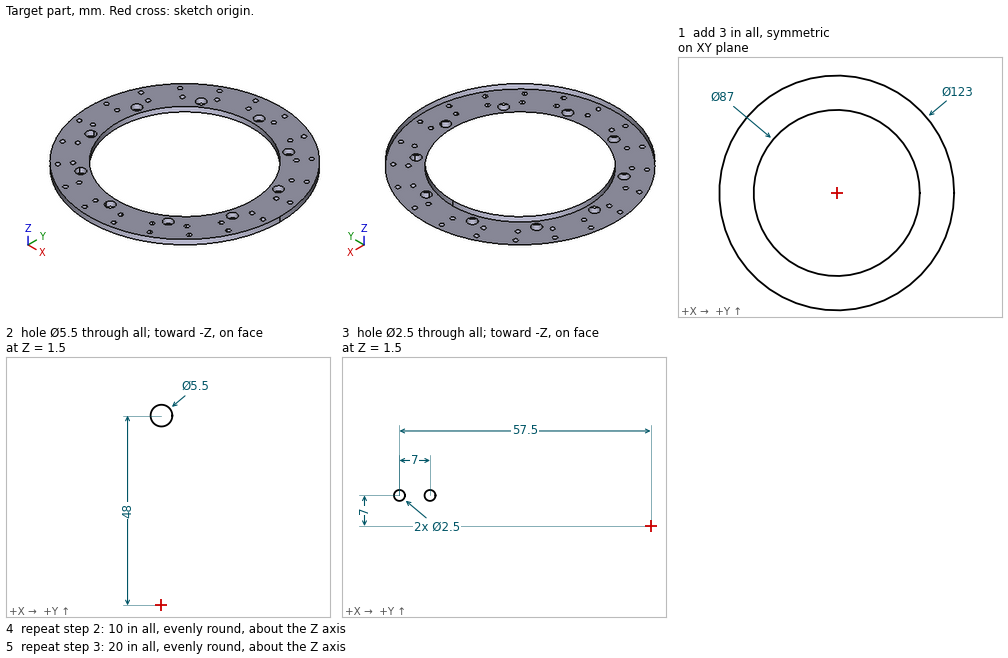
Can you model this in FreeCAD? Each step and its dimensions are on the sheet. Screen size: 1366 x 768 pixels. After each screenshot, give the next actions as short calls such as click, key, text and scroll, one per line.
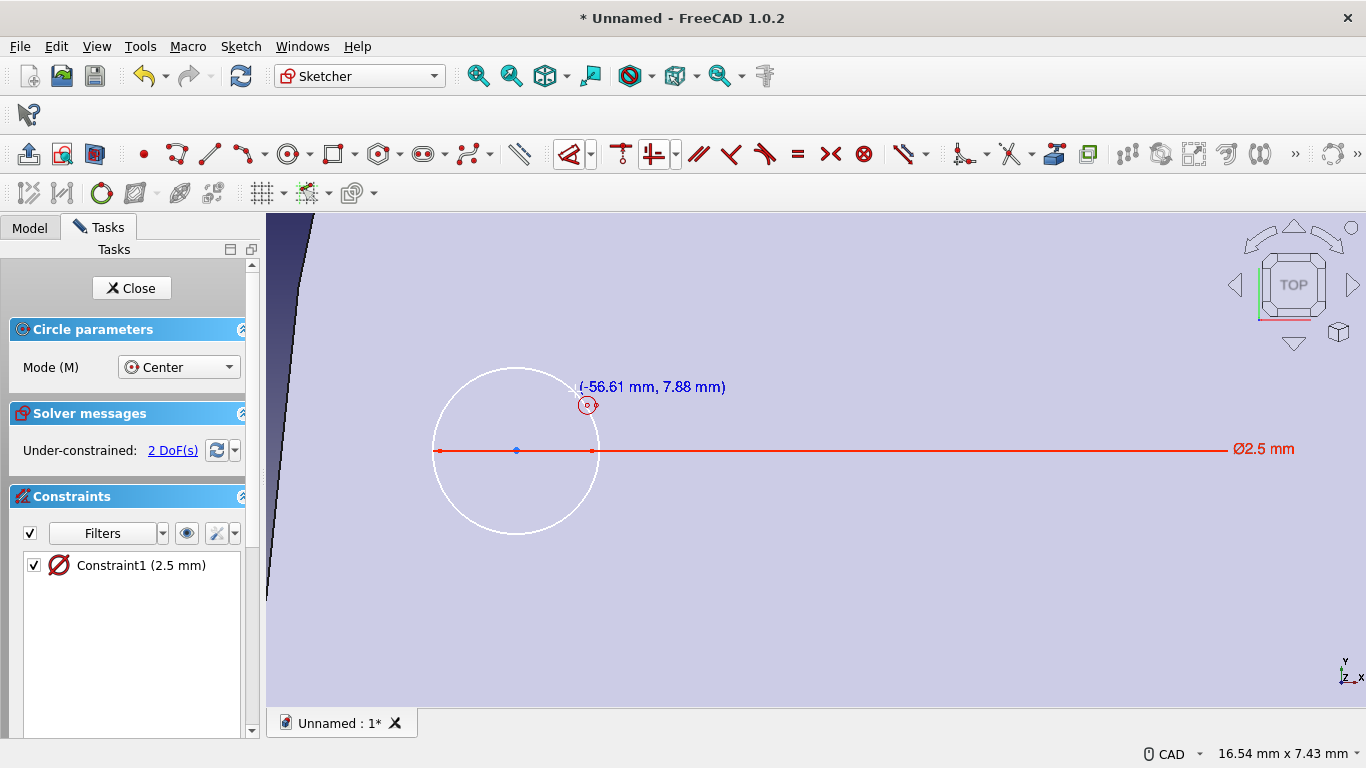
click(981, 450)
move(1040, 391)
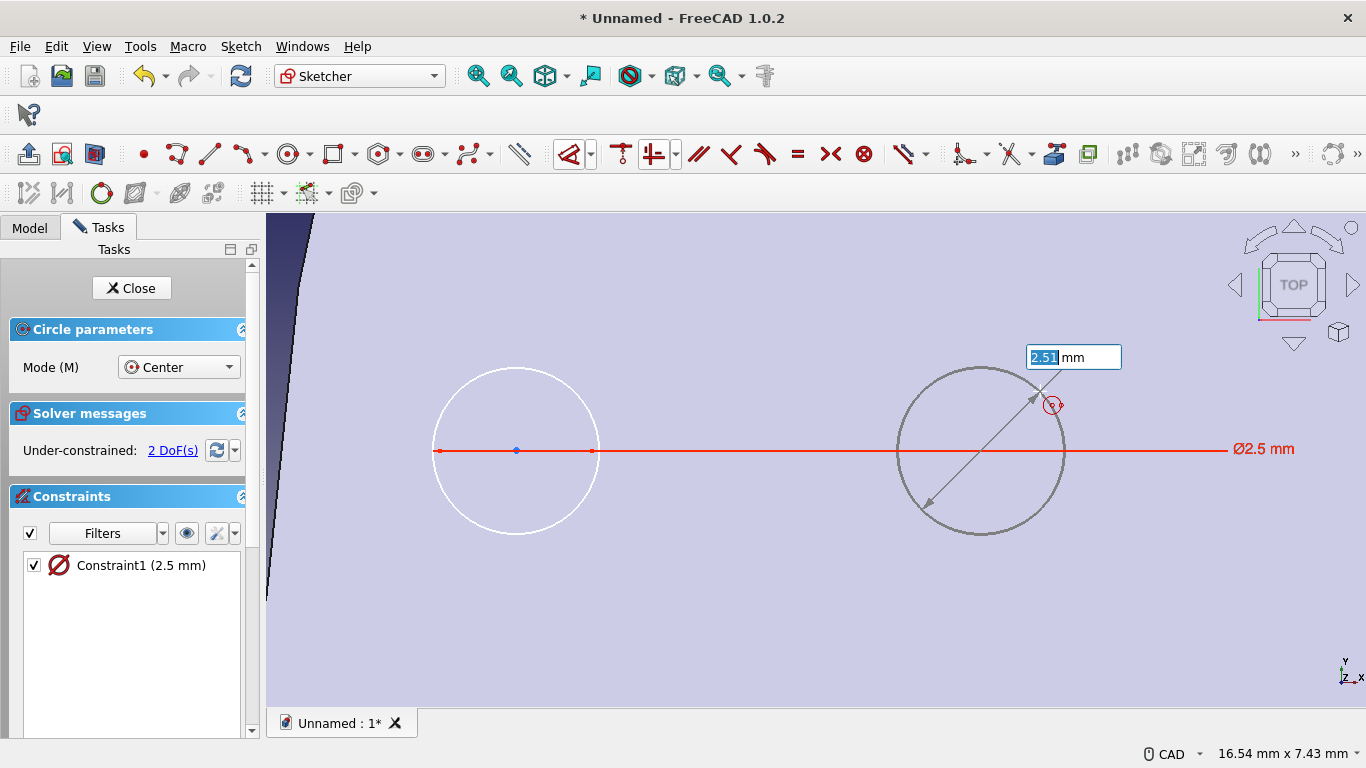
text(2.5)
key(Return)
key(Escape)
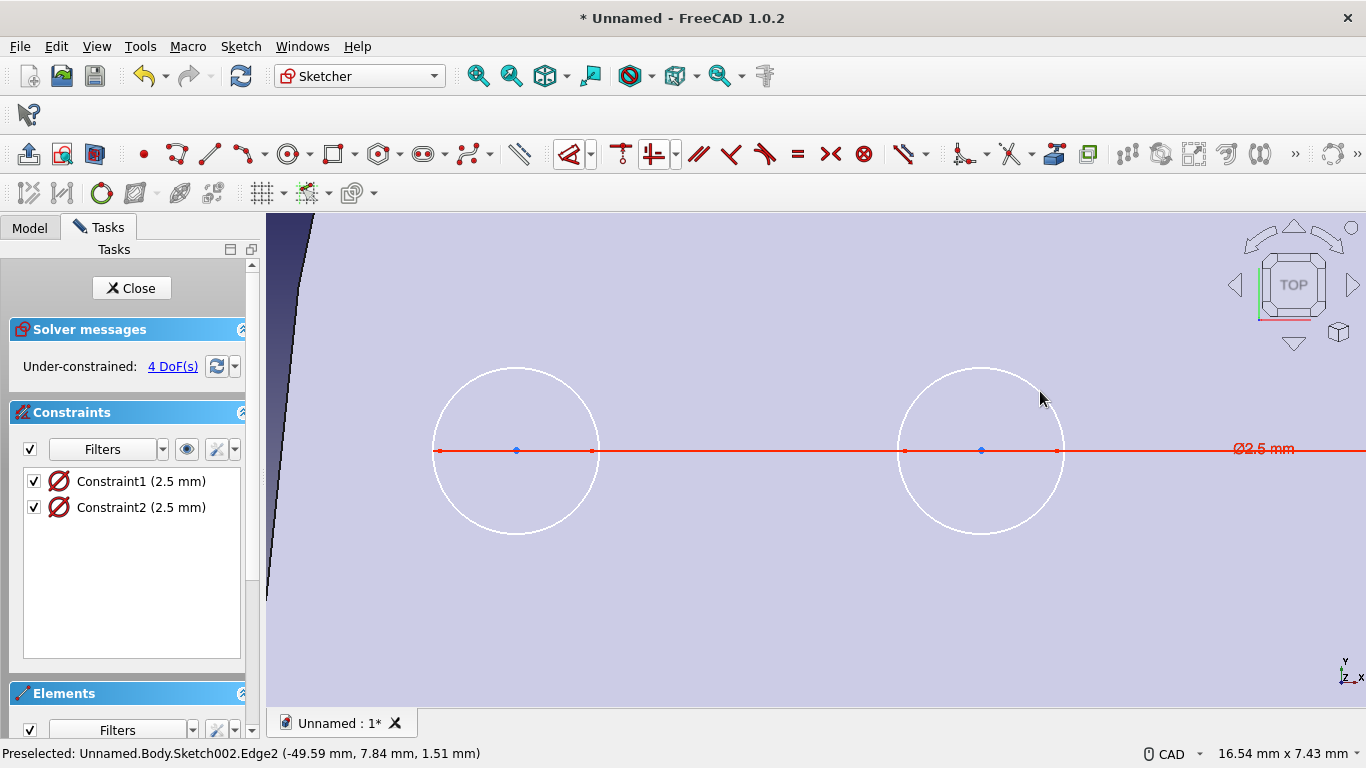
click(516, 451)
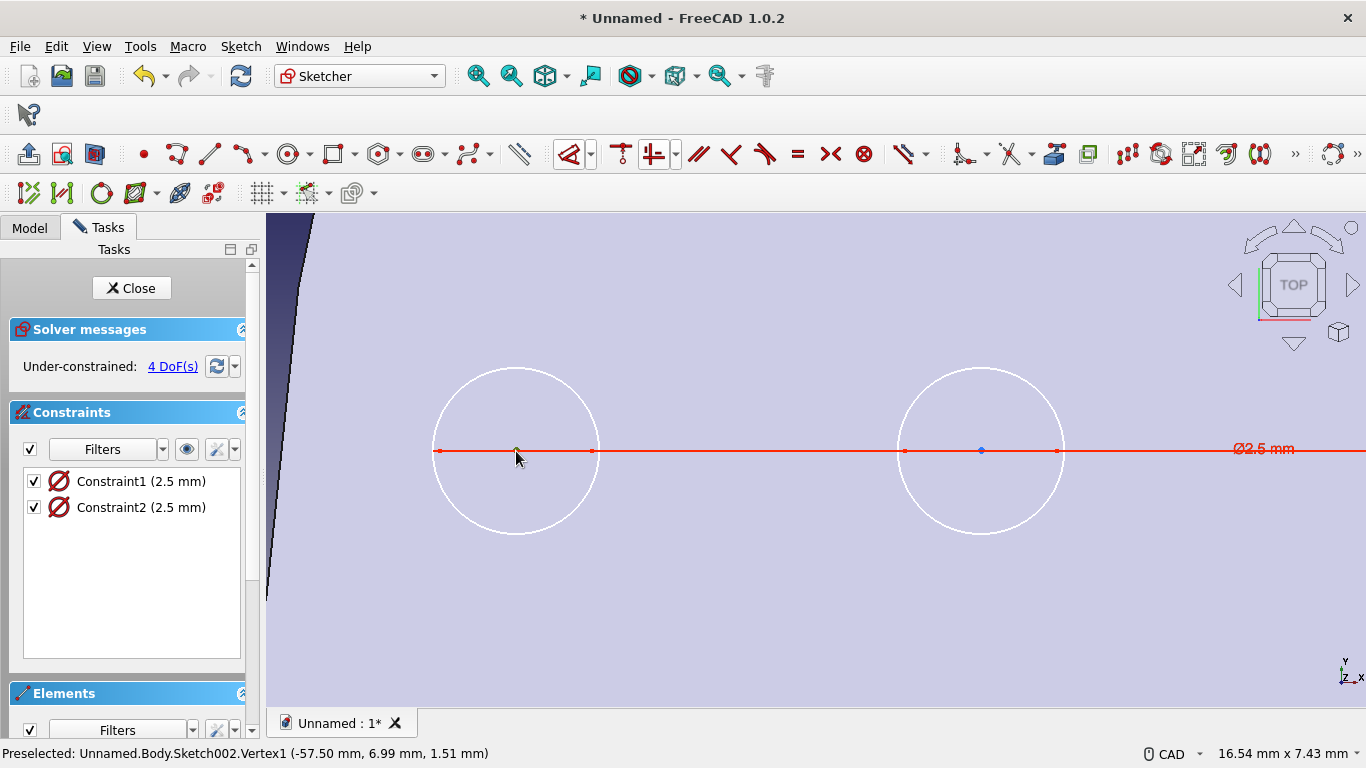
click(981, 451)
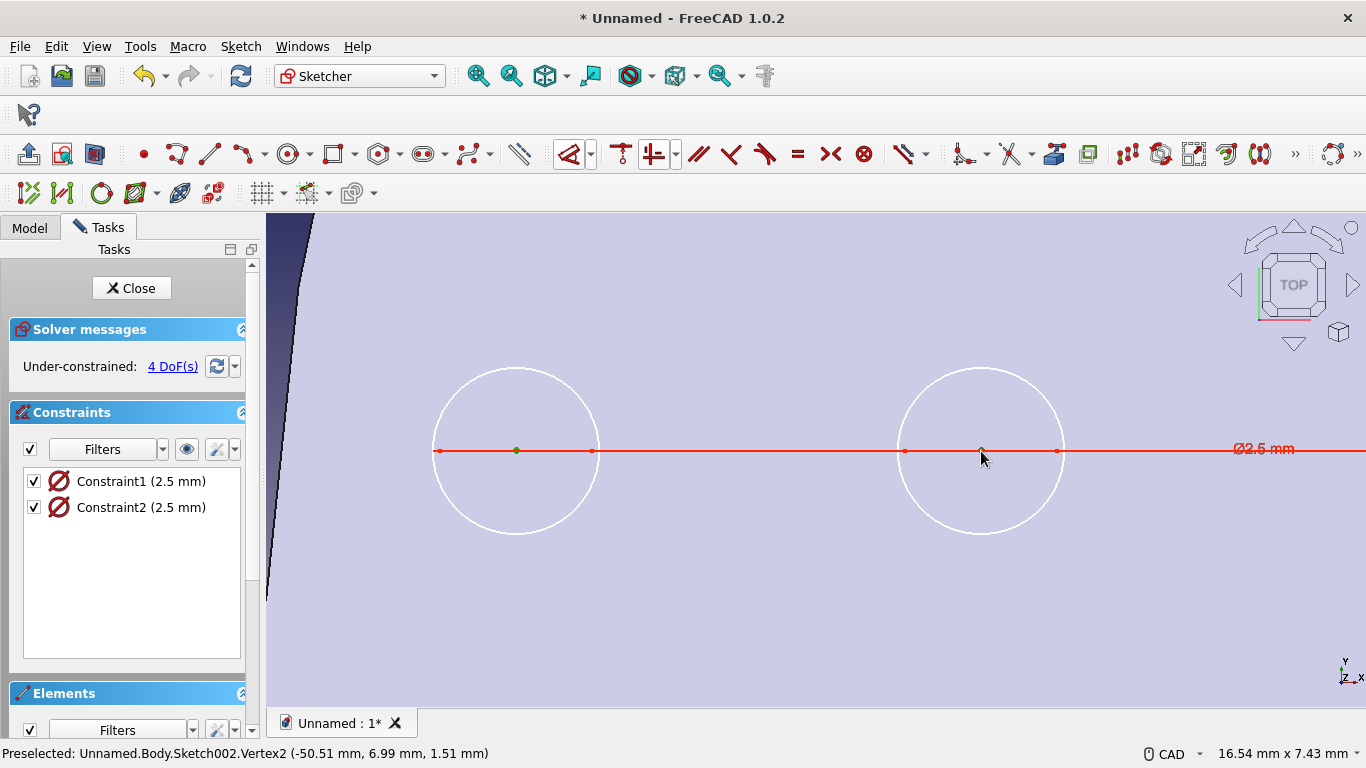
key(h)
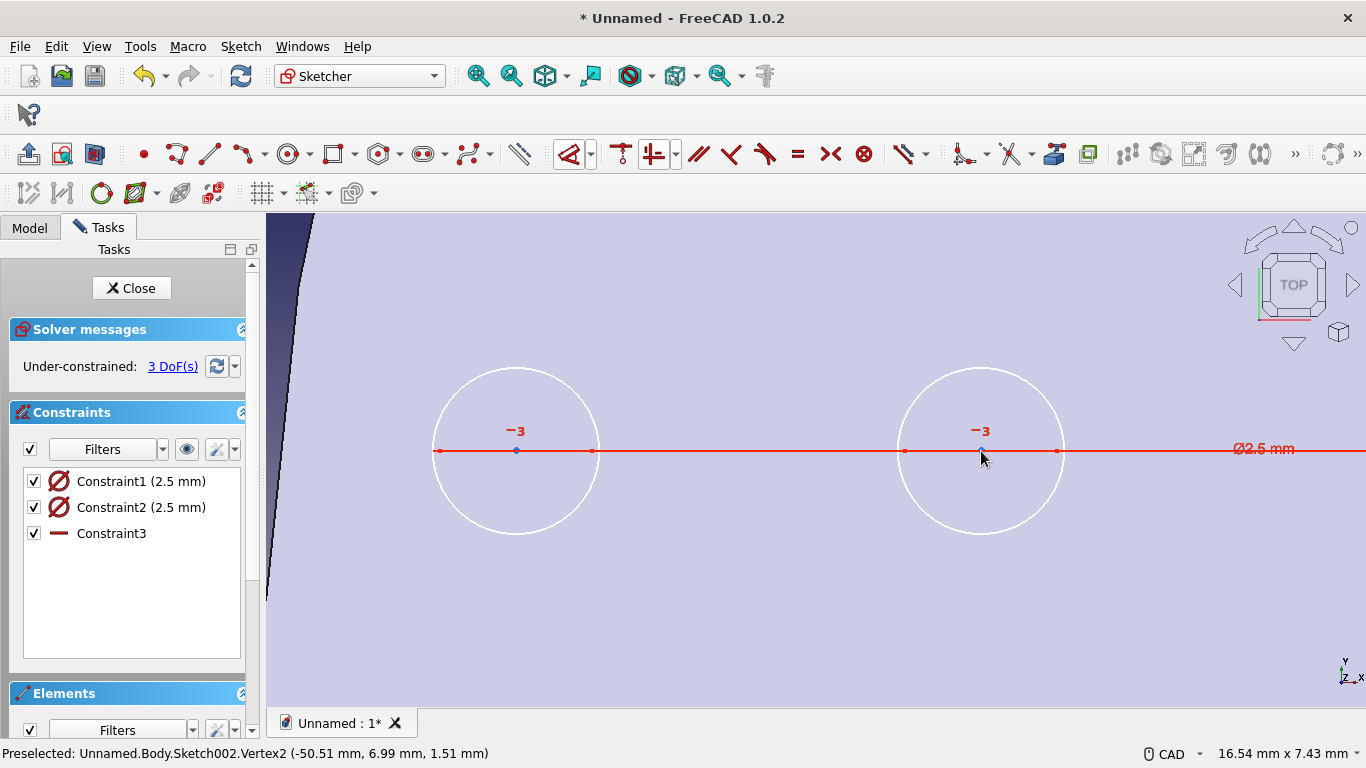
click(516, 451)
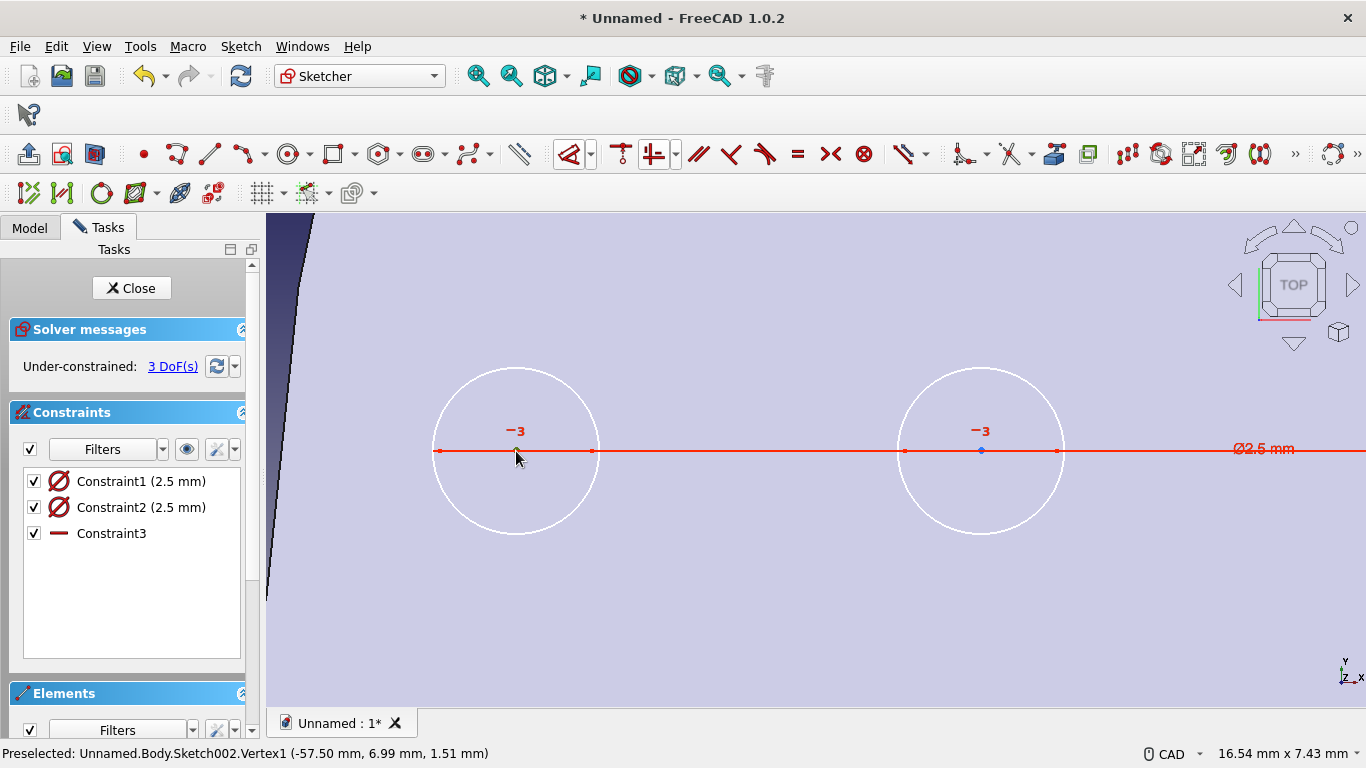
key(i)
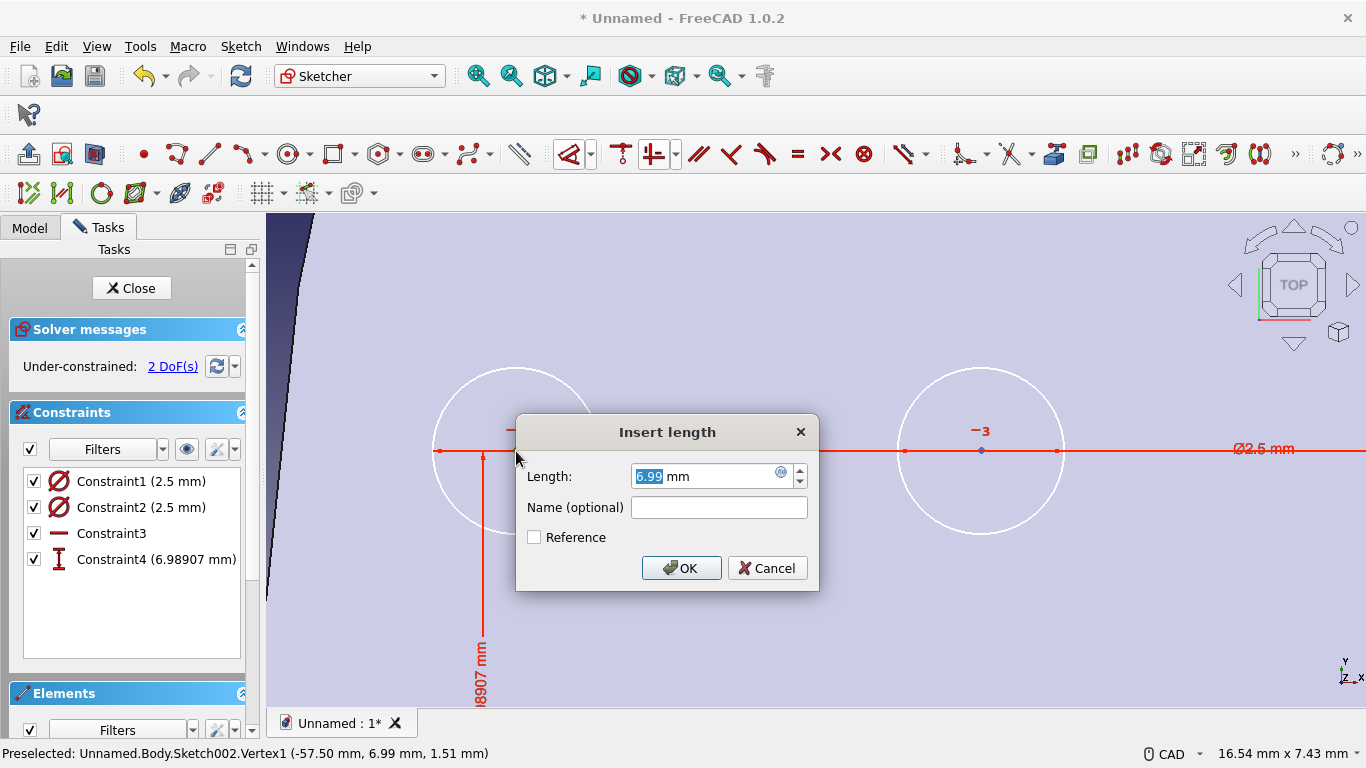
text(7)
key(Return)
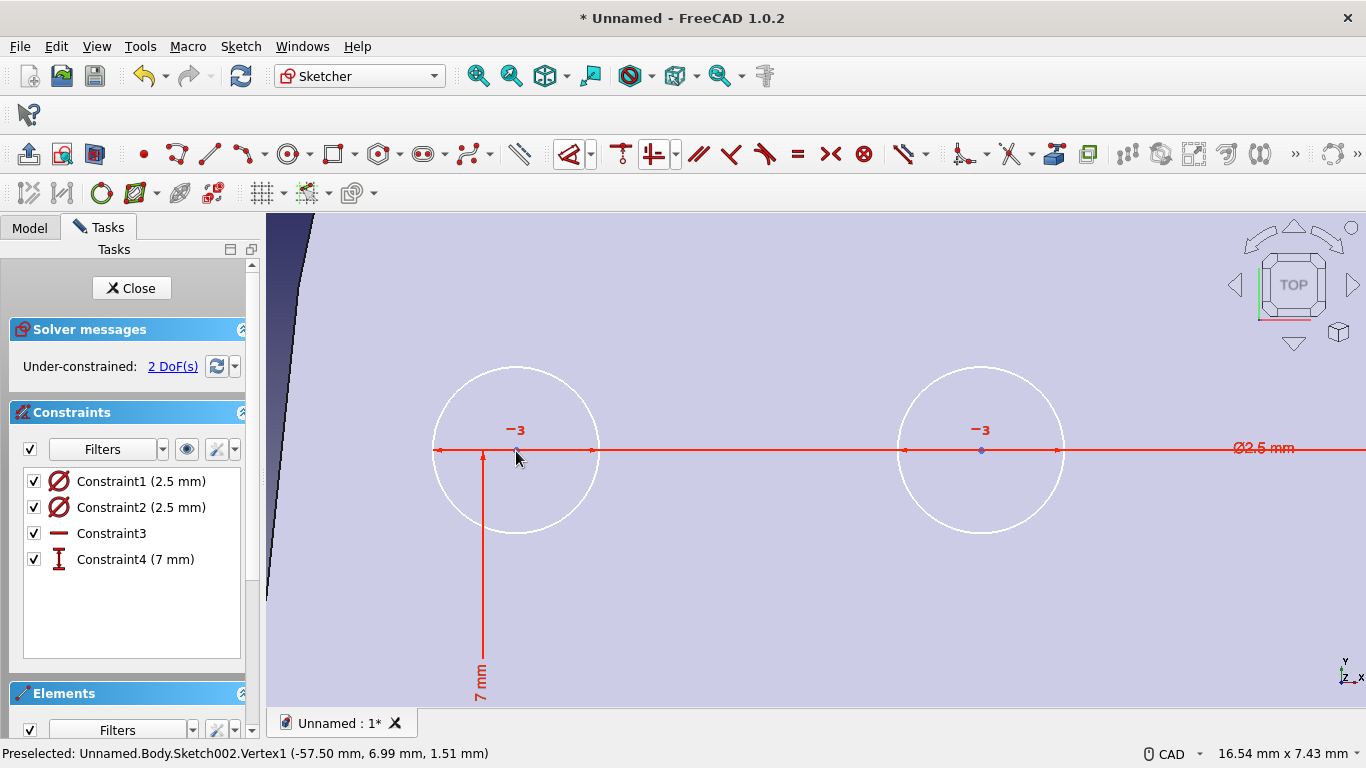
click(516, 450)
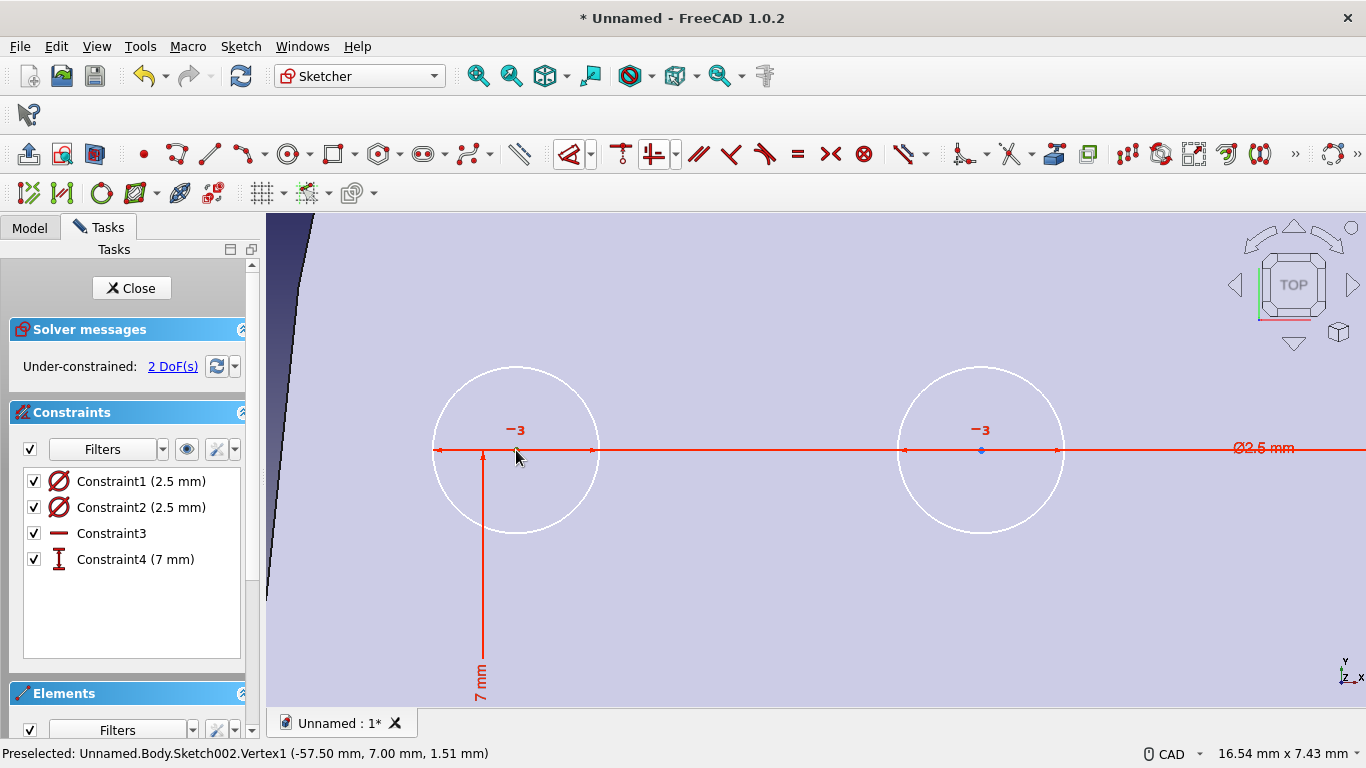
click(981, 450)